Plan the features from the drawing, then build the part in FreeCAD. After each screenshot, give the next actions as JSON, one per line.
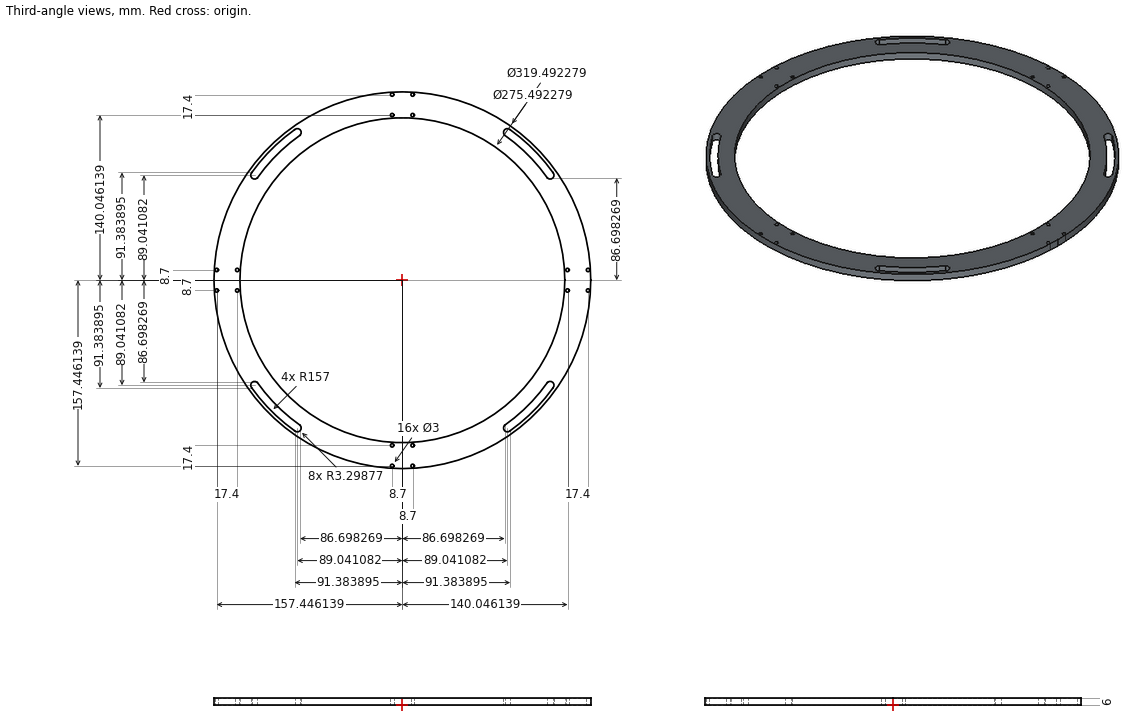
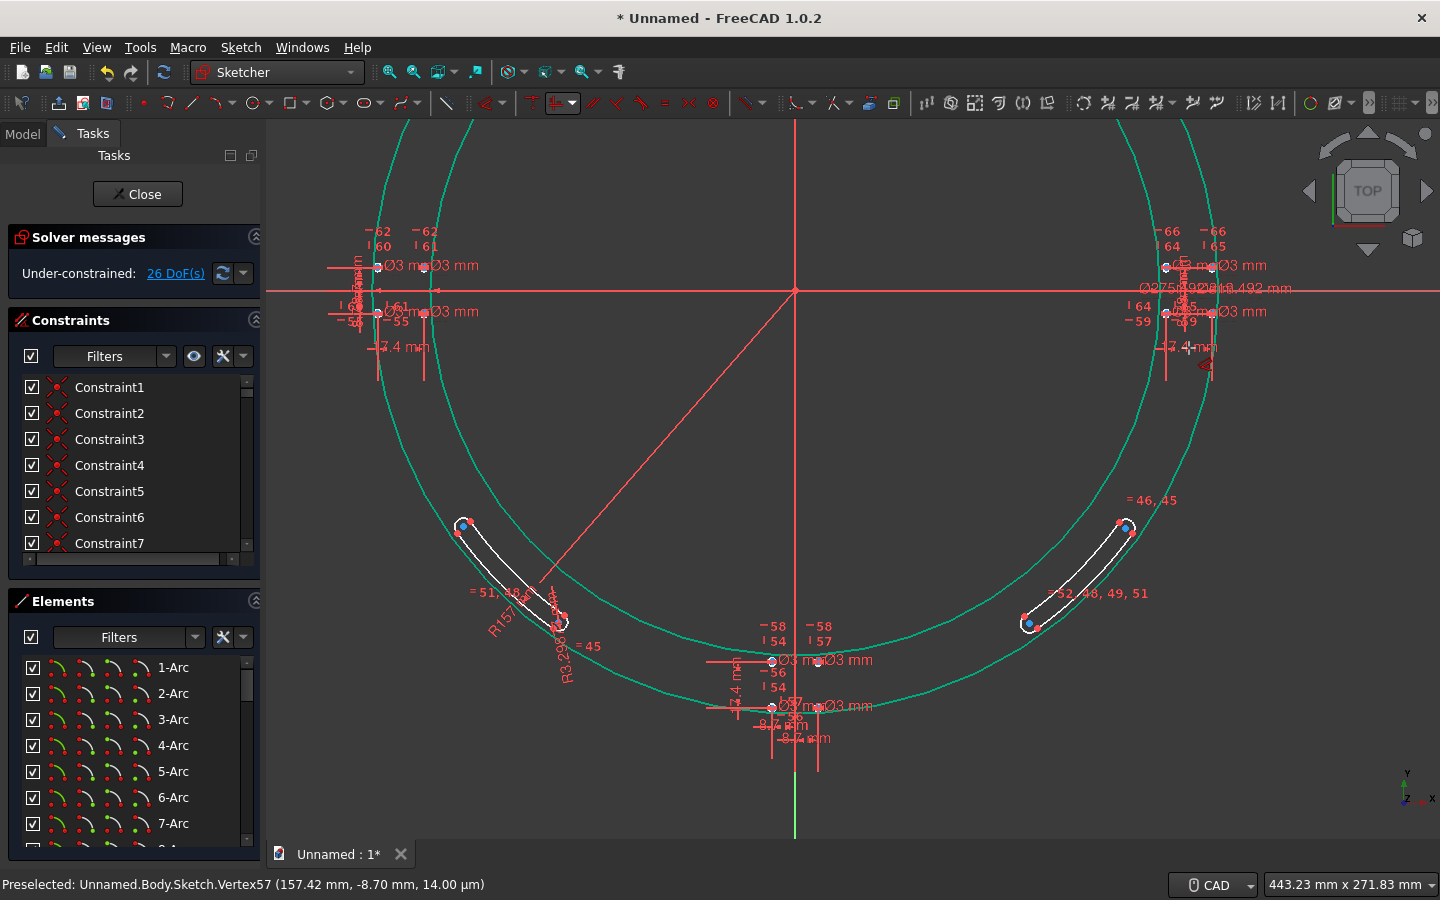
{"action": "scroll", "coordinate": [771, 708], "scroll_direction": "down", "scroll_amount": 3}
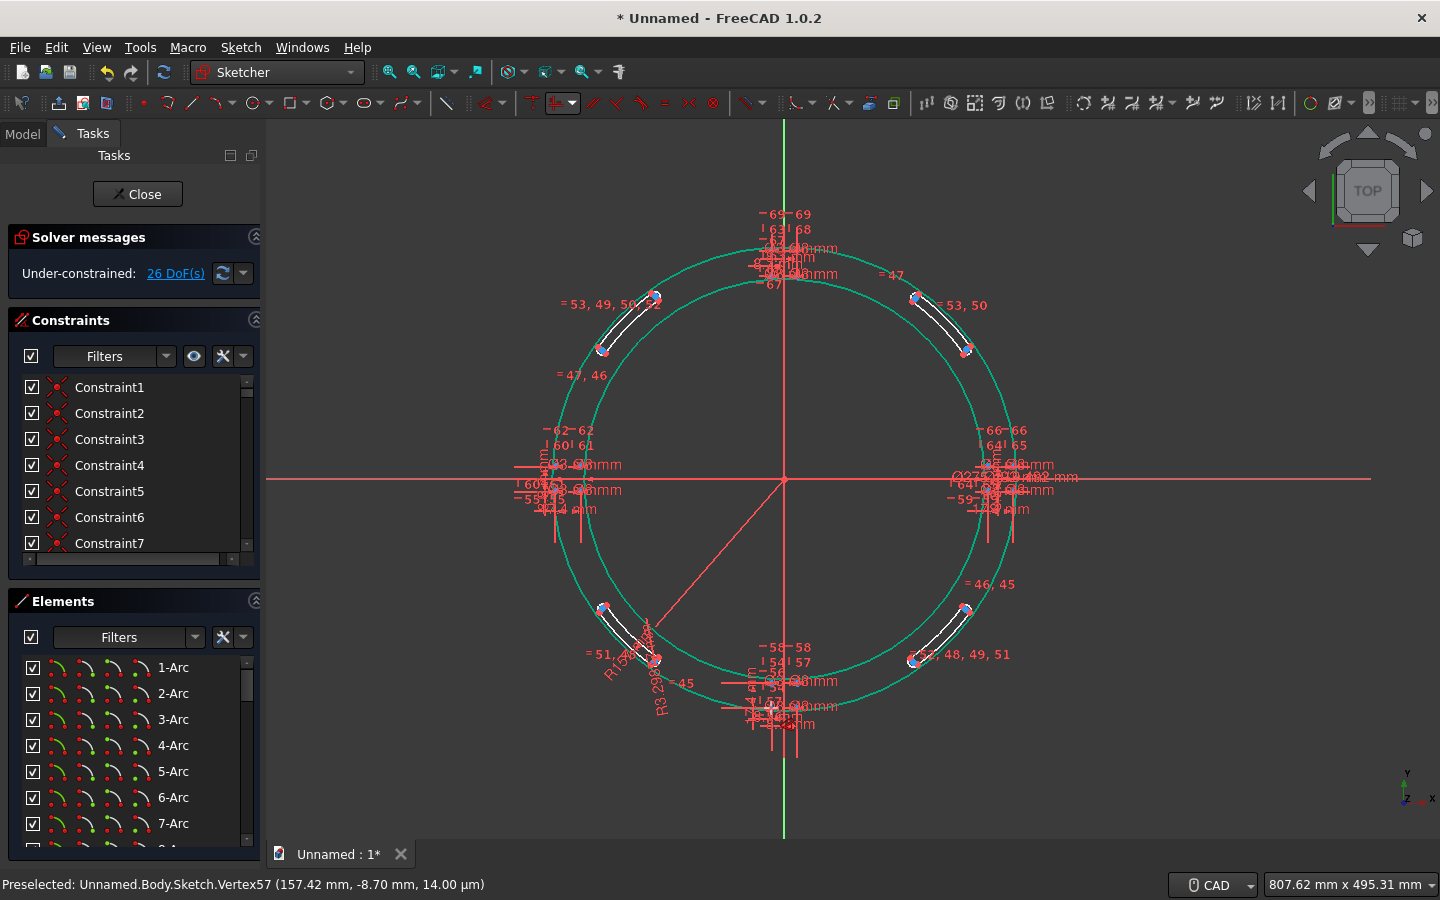
{"action": "scroll", "coordinate": [772, 276], "scroll_direction": "up", "scroll_amount": 3}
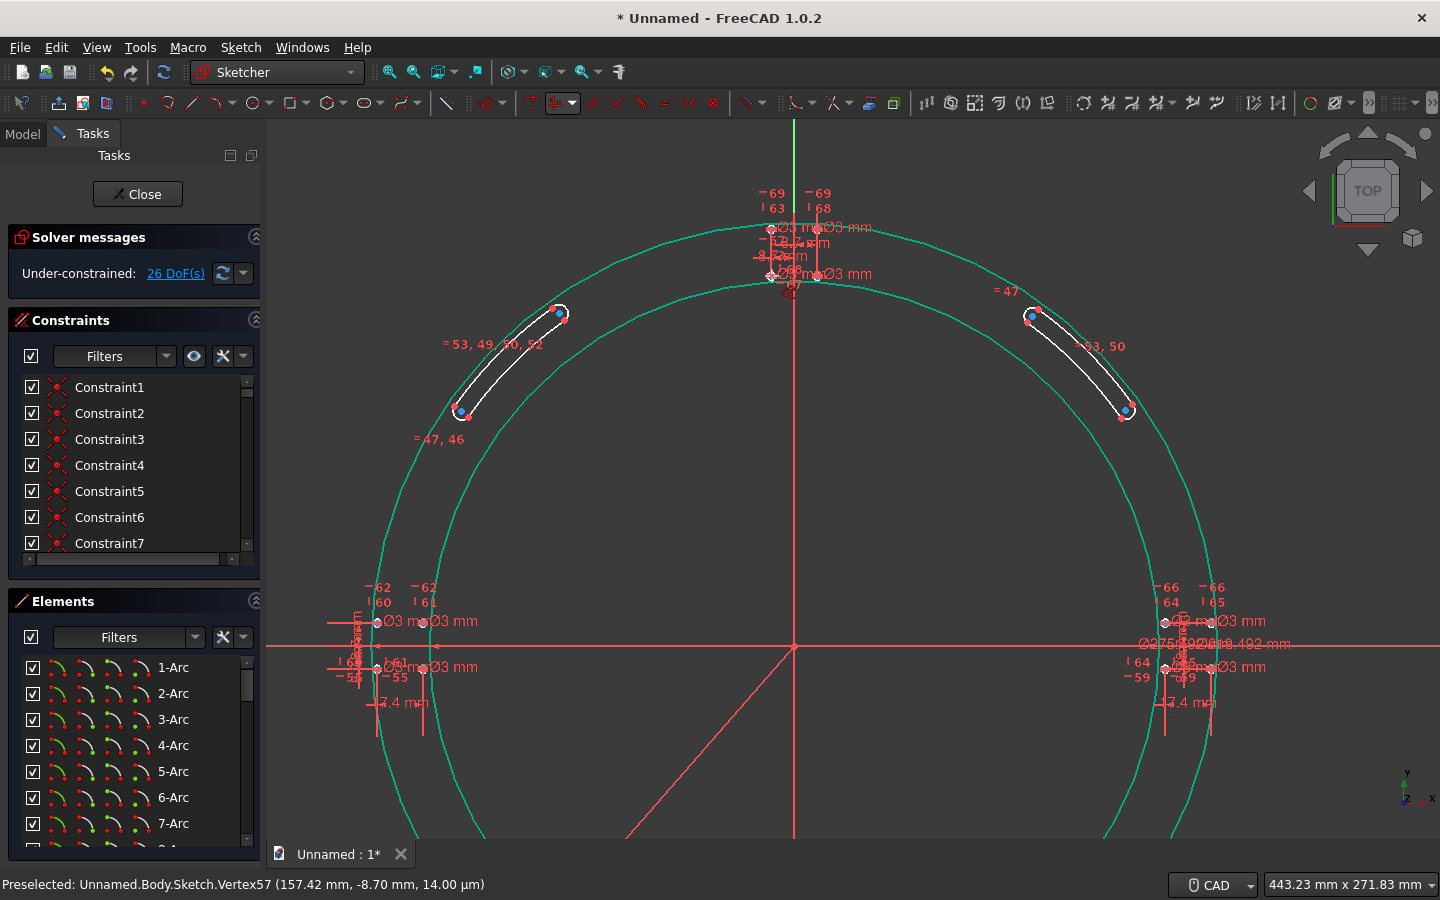
{"action": "left_click", "coordinate": [771, 276]}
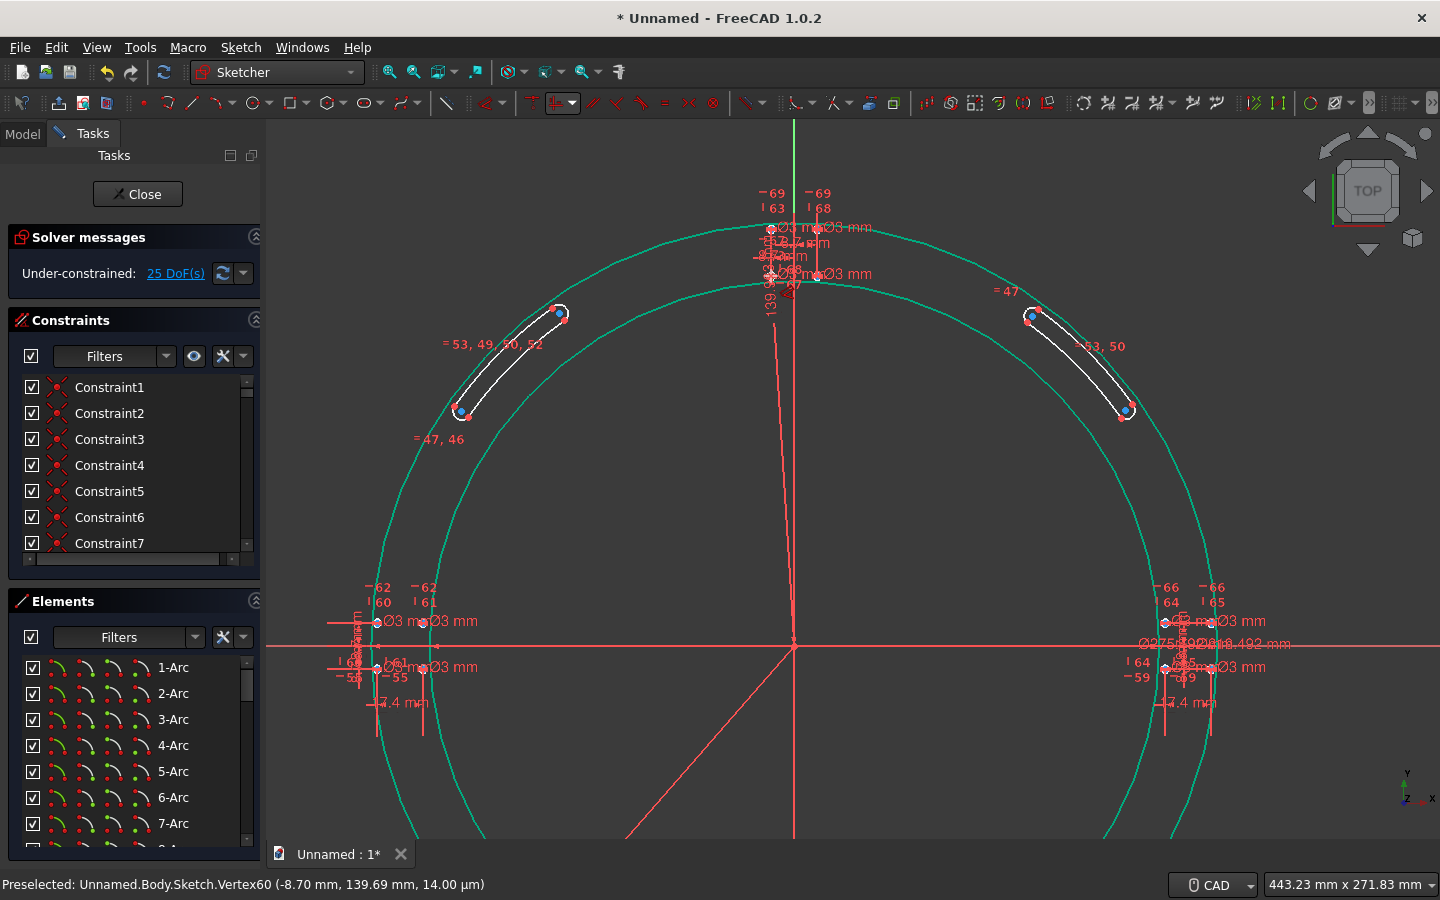
{"action": "left_click", "coordinate": [771, 229]}
{"action": "left_click", "coordinate": [689, 253]}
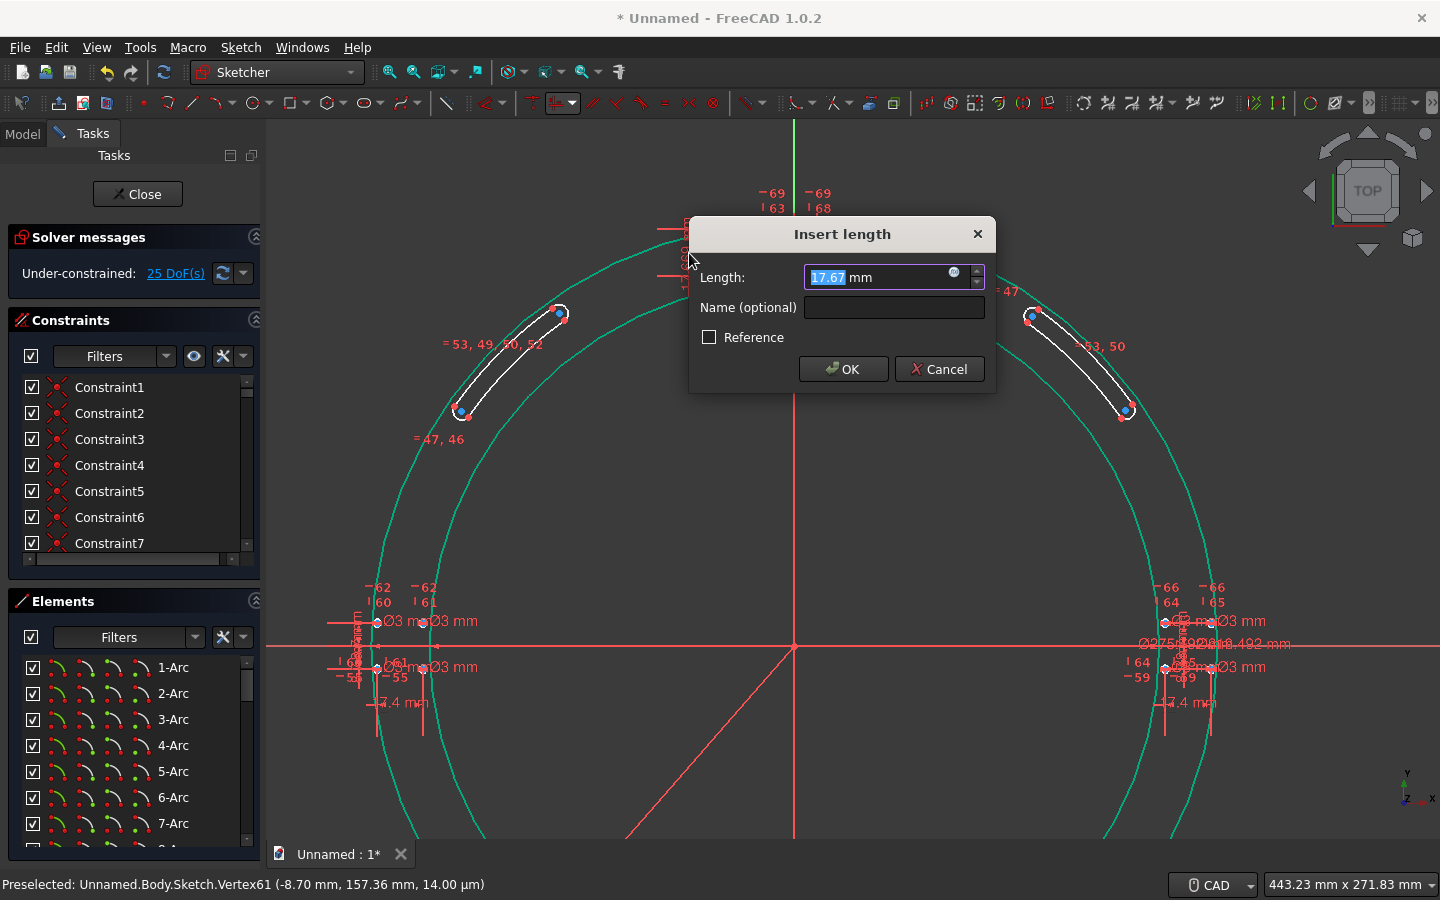
{"action": "type", "text": "17.4"}
{"action": "key", "text": "Return"}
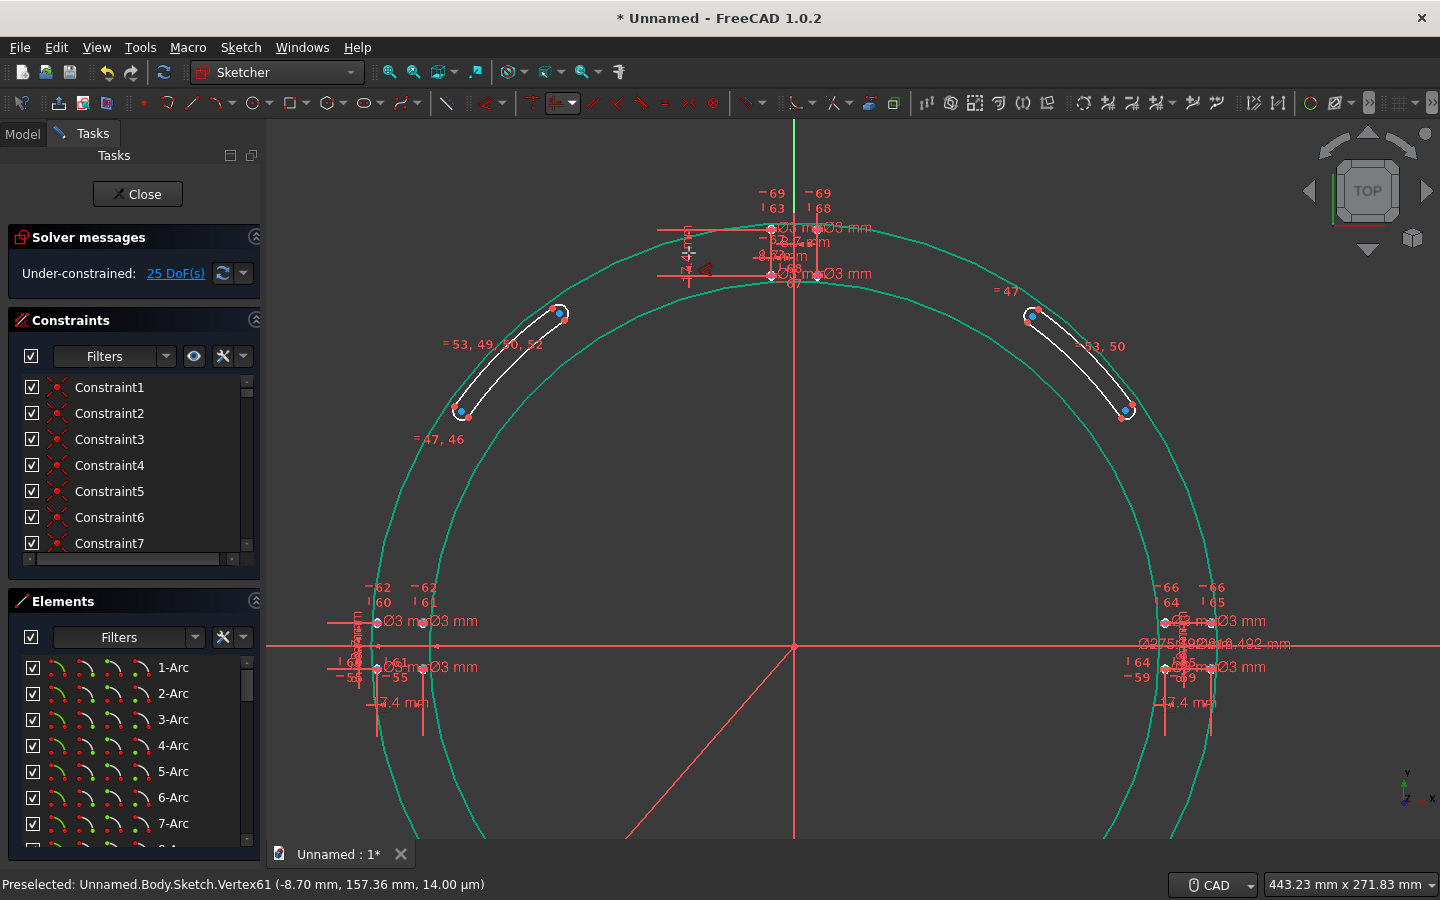
{"action": "scroll", "coordinate": [772, 276], "scroll_direction": "down", "scroll_amount": 3}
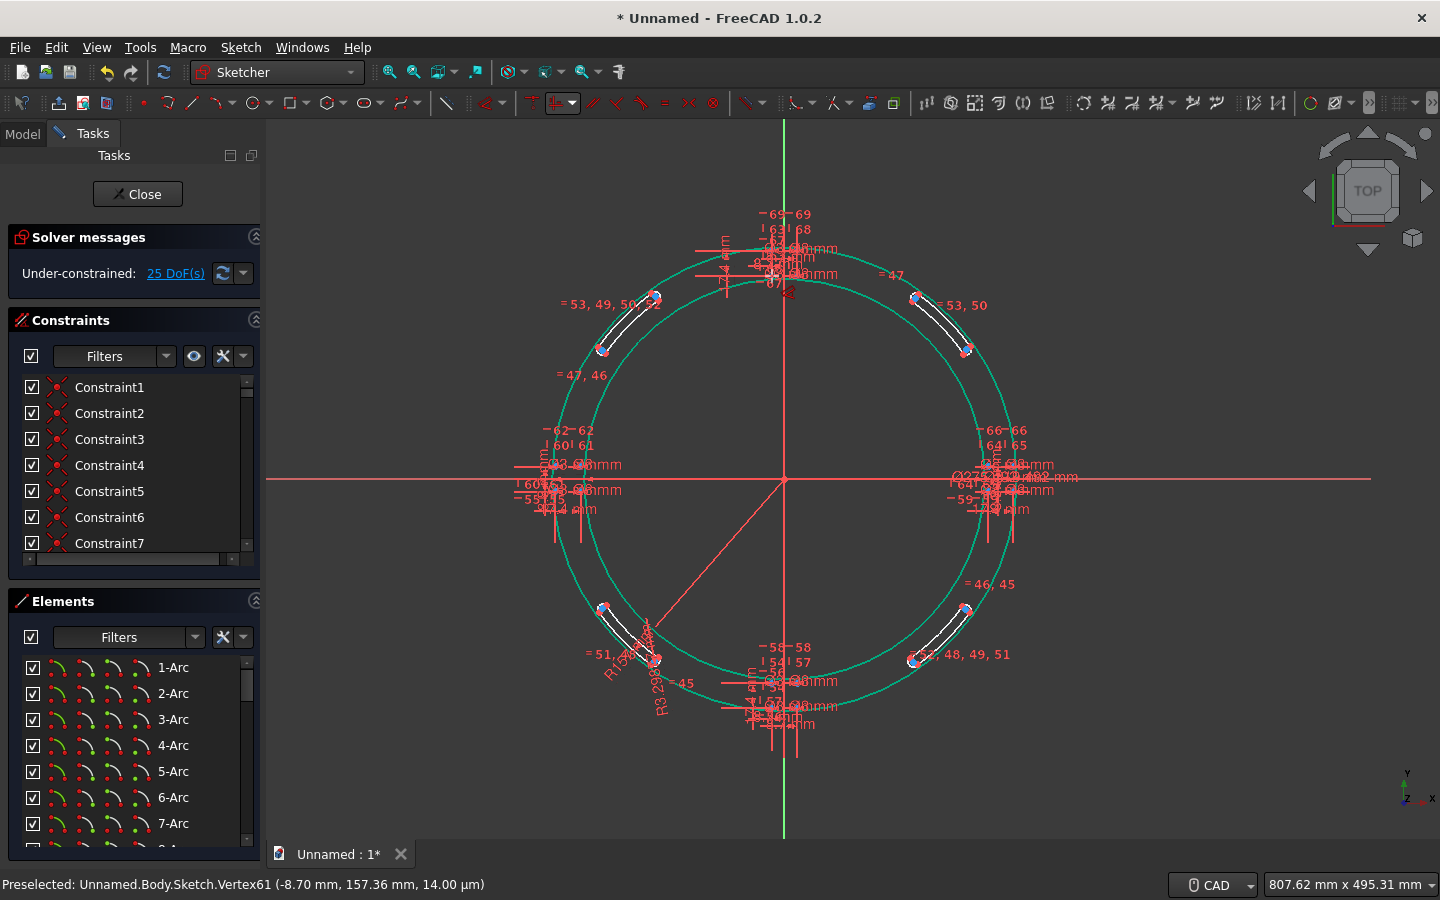
{"action": "scroll", "coordinate": [652, 665], "scroll_direction": "up", "scroll_amount": 5}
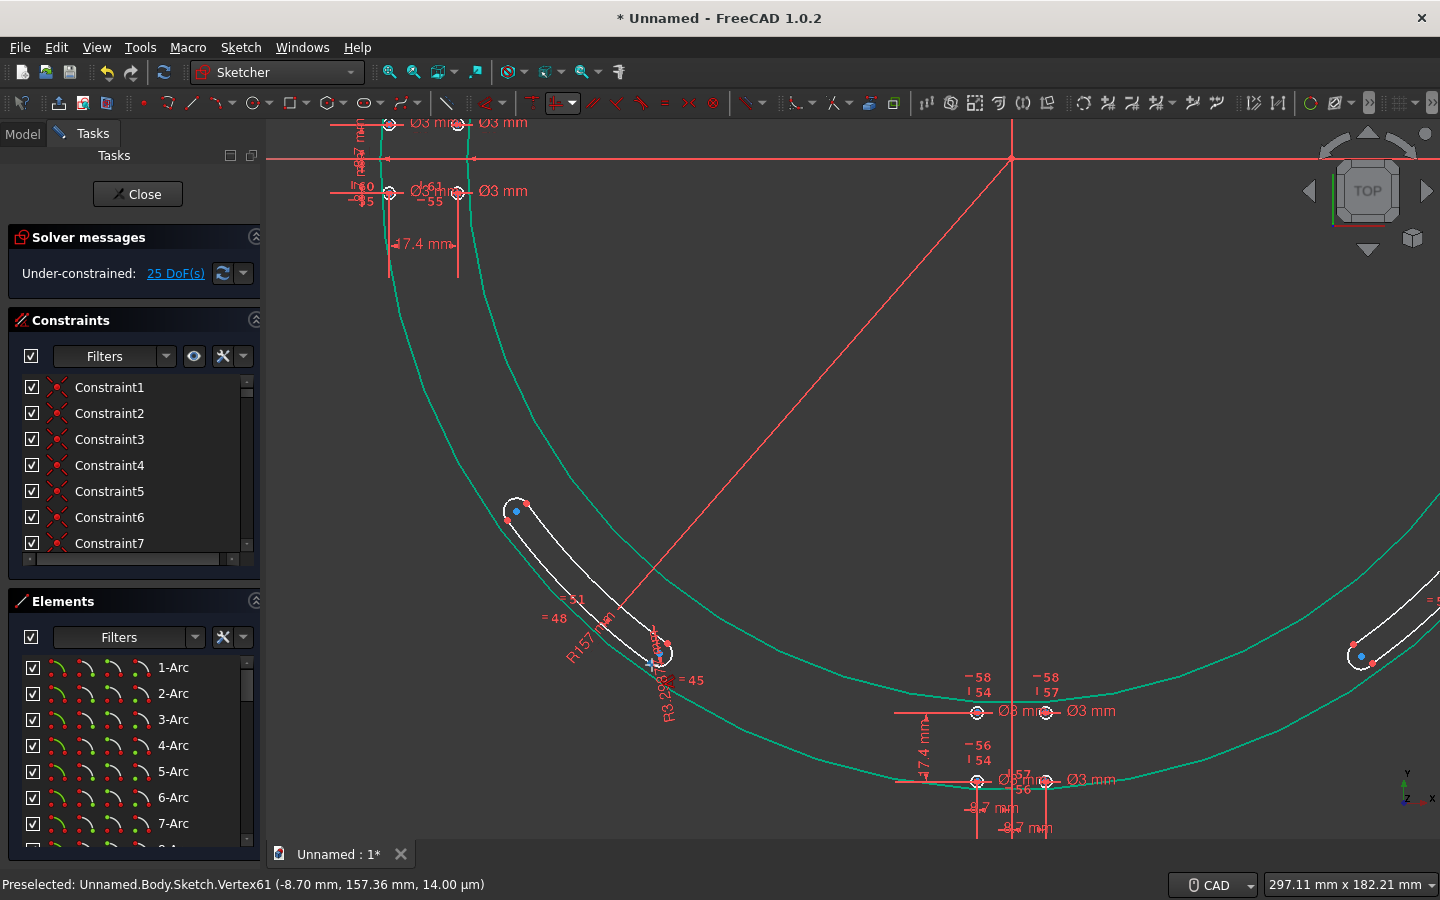
{"action": "left_click", "coordinate": [651, 664]}
{"action": "left_click", "coordinate": [831, 698]}